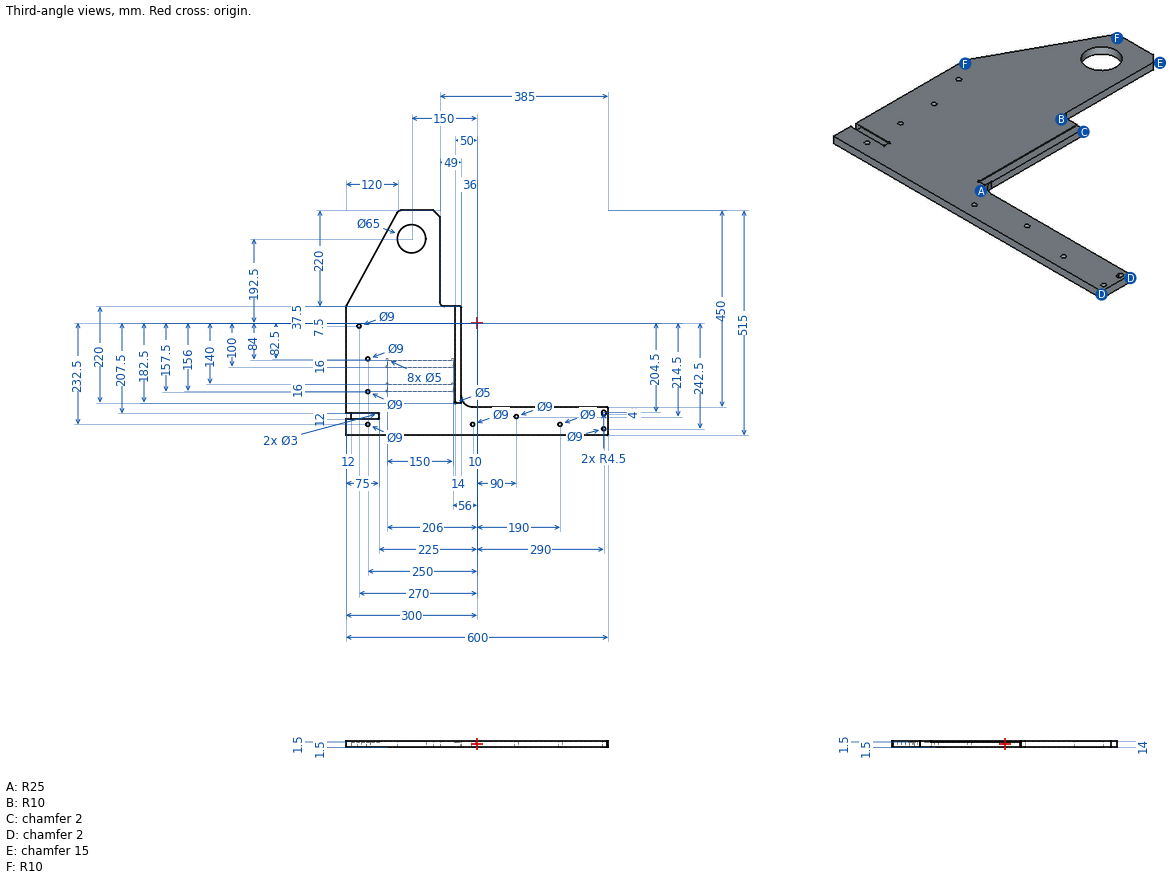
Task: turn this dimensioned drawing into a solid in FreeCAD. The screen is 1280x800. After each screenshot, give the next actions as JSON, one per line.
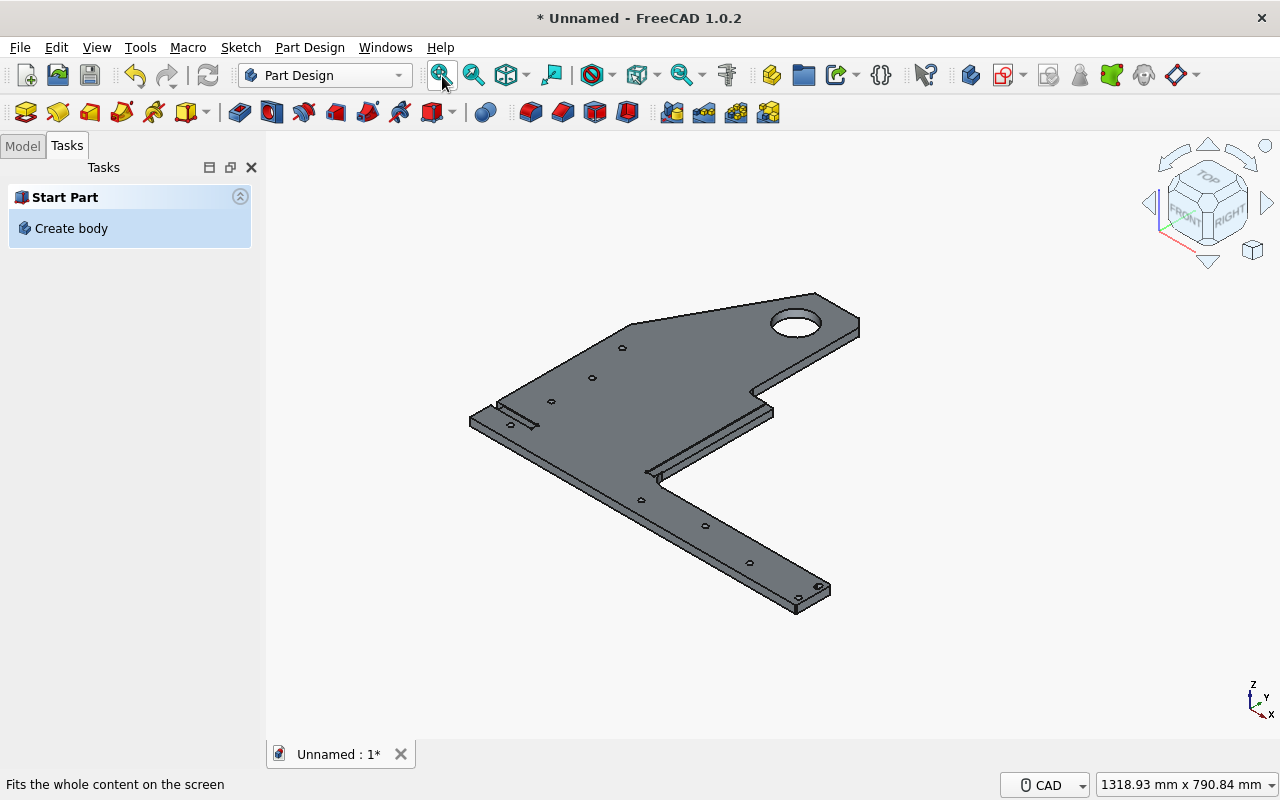
{"action": "key", "text": "2"}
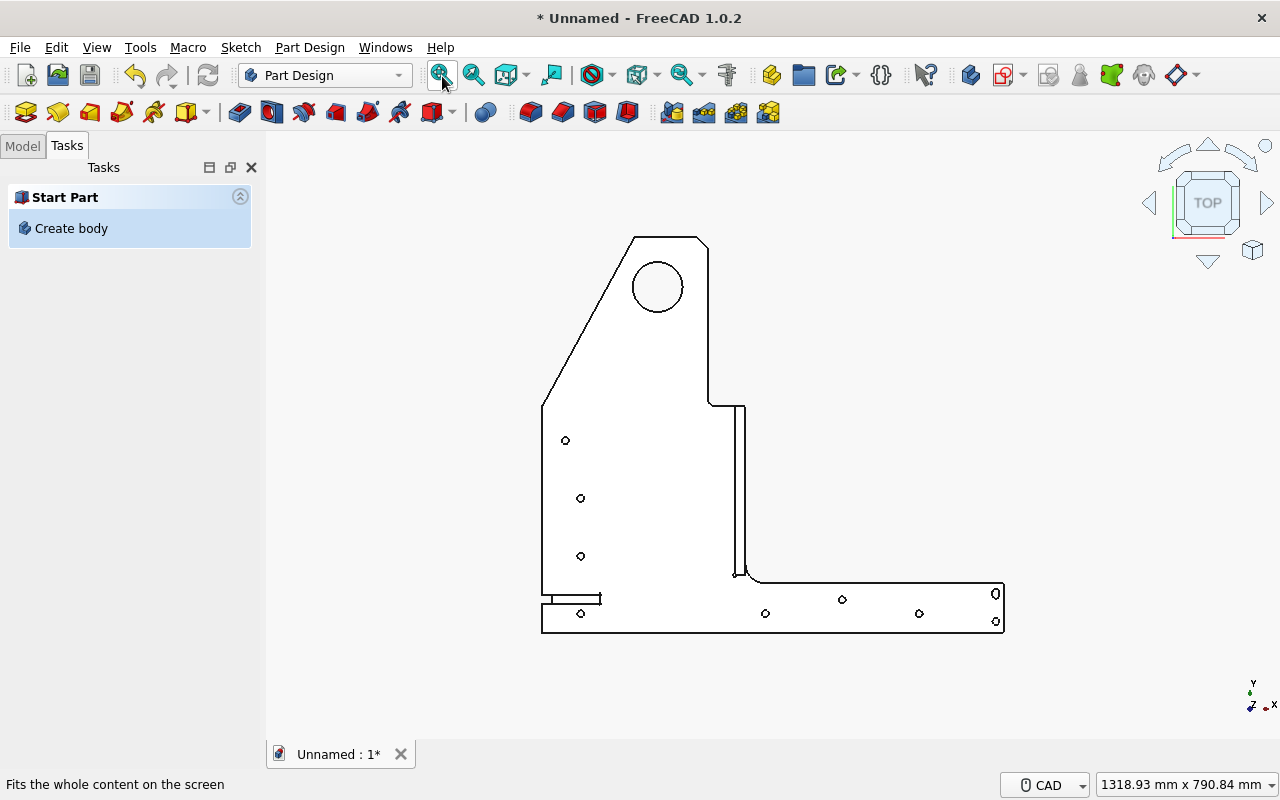
{"action": "scroll", "coordinate": [635, 236], "scroll_direction": "up", "scroll_amount": 7}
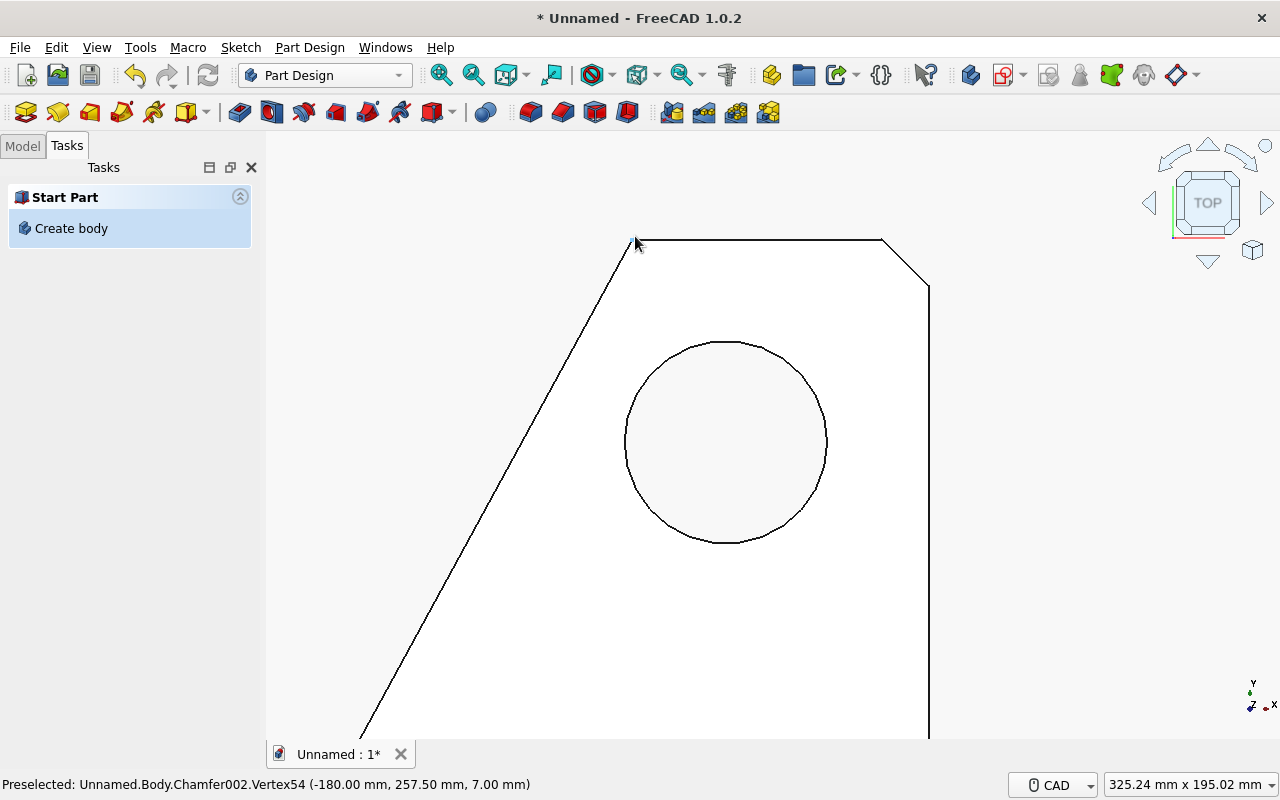
{"action": "left_click", "coordinate": [442, 76]}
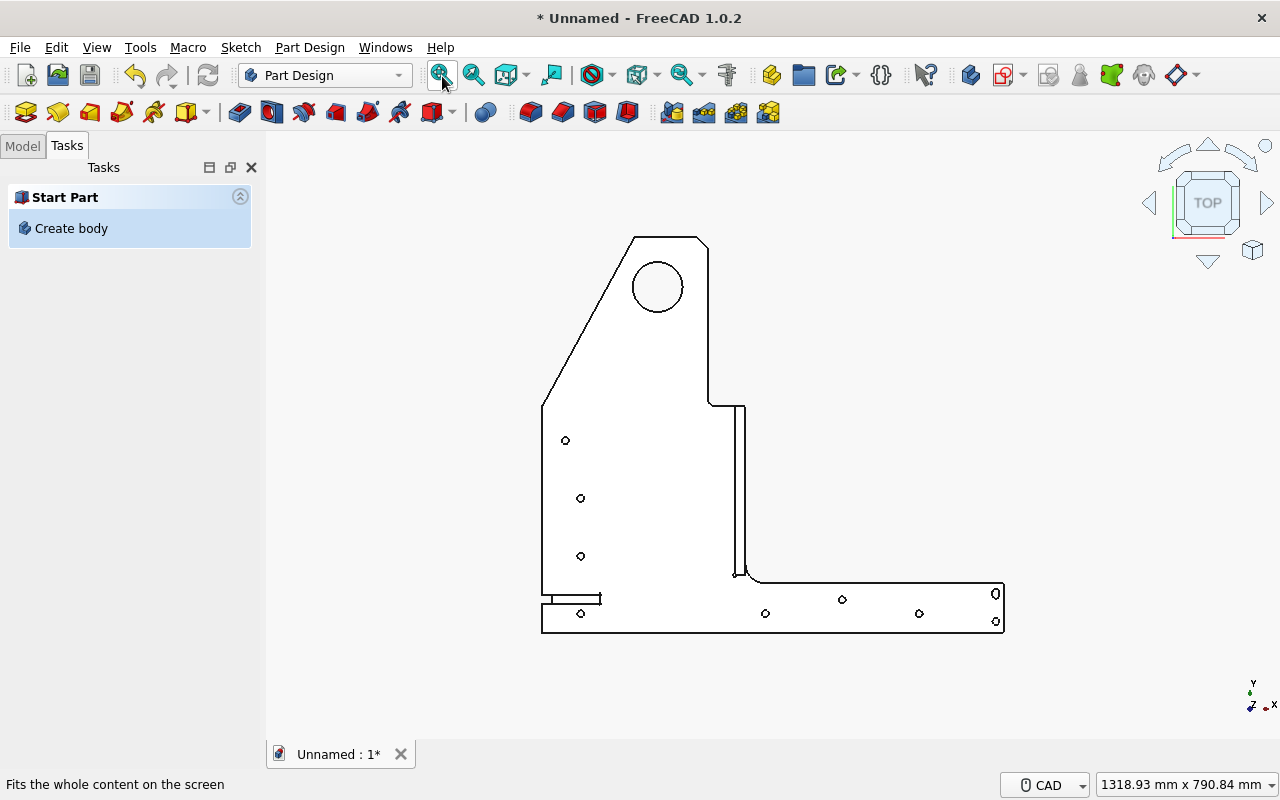
{"action": "key", "text": "1"}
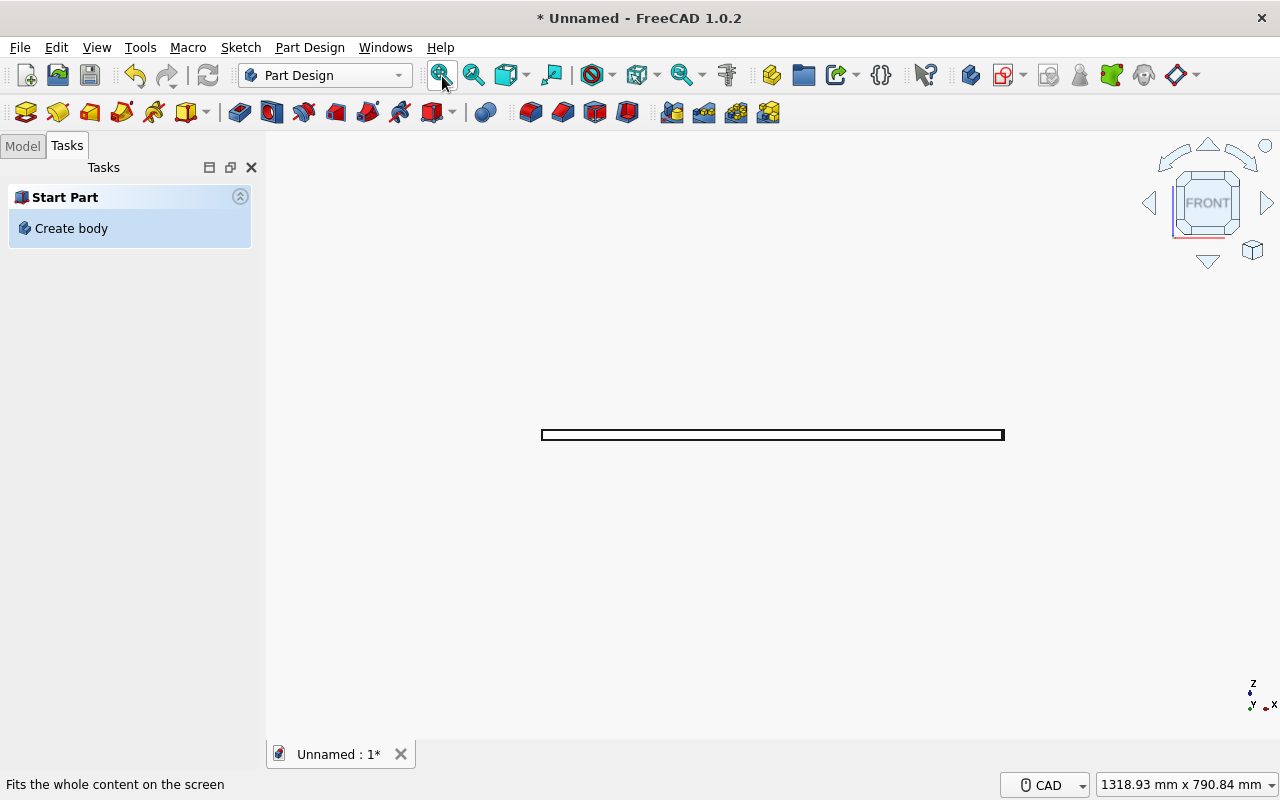
{"action": "scroll", "coordinate": [635, 434], "scroll_direction": "up", "scroll_amount": 7}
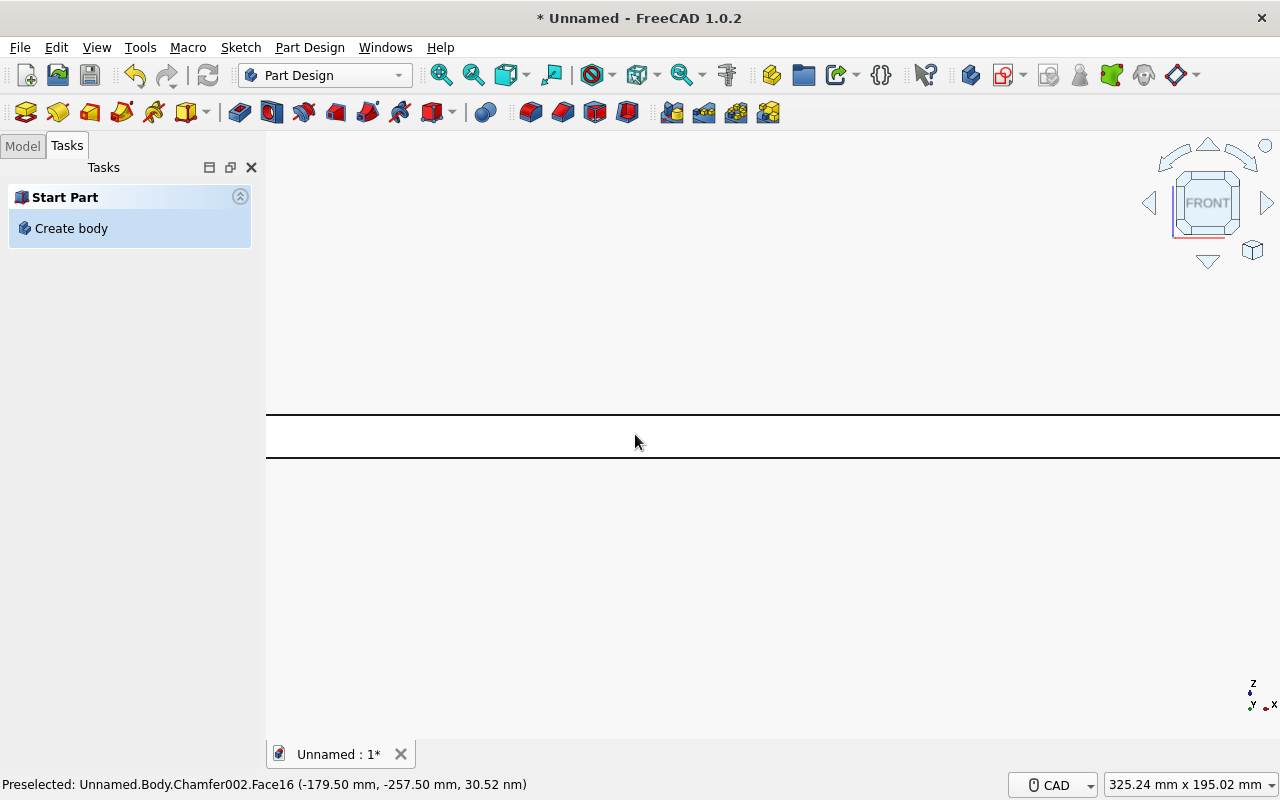
{"action": "left_click", "coordinate": [442, 76]}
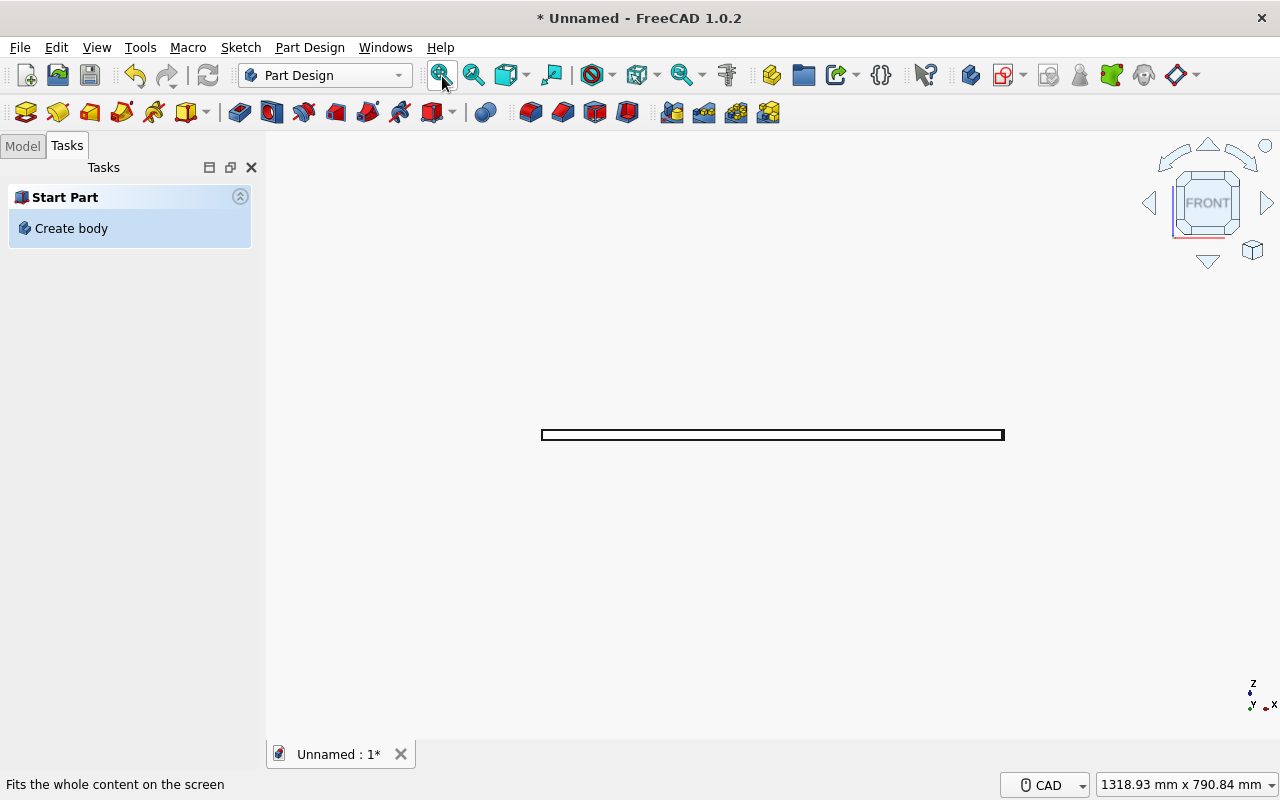
{"action": "key", "text": "3"}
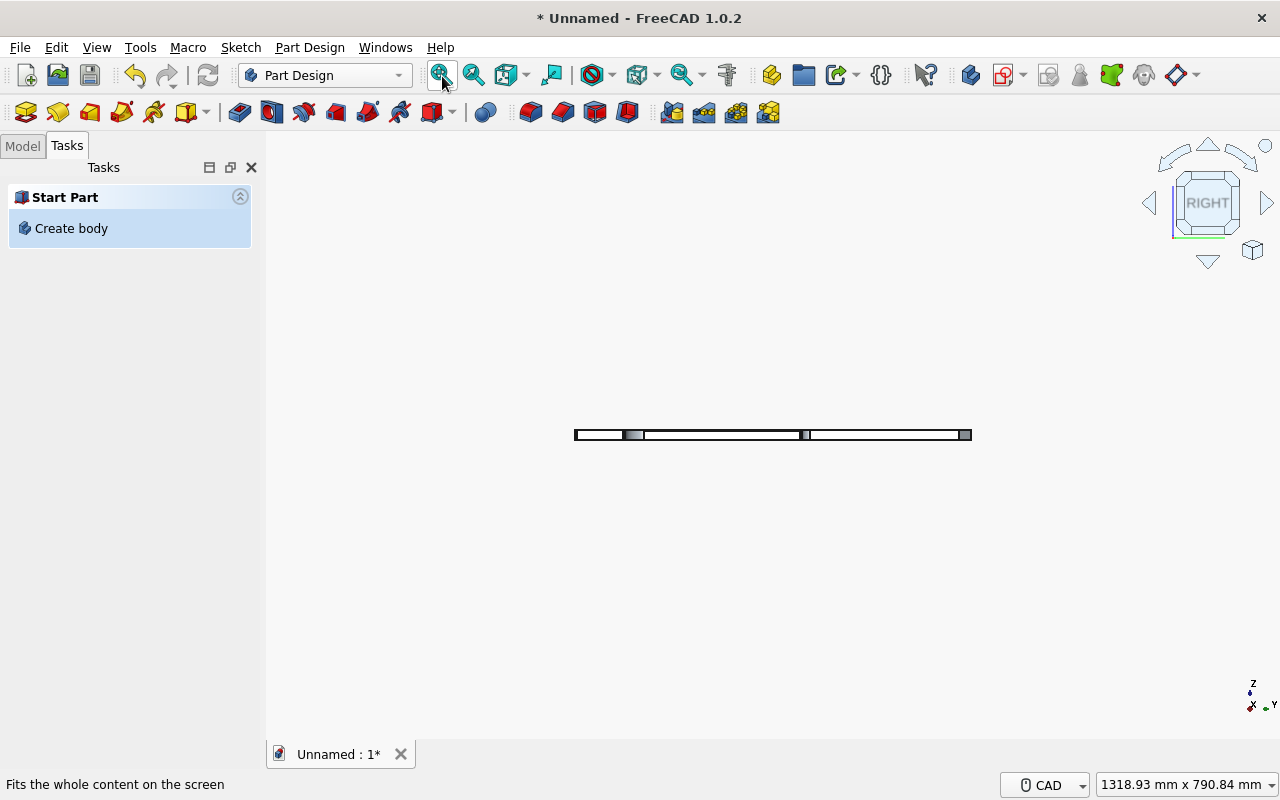
{"action": "left_click", "coordinate": [442, 76]}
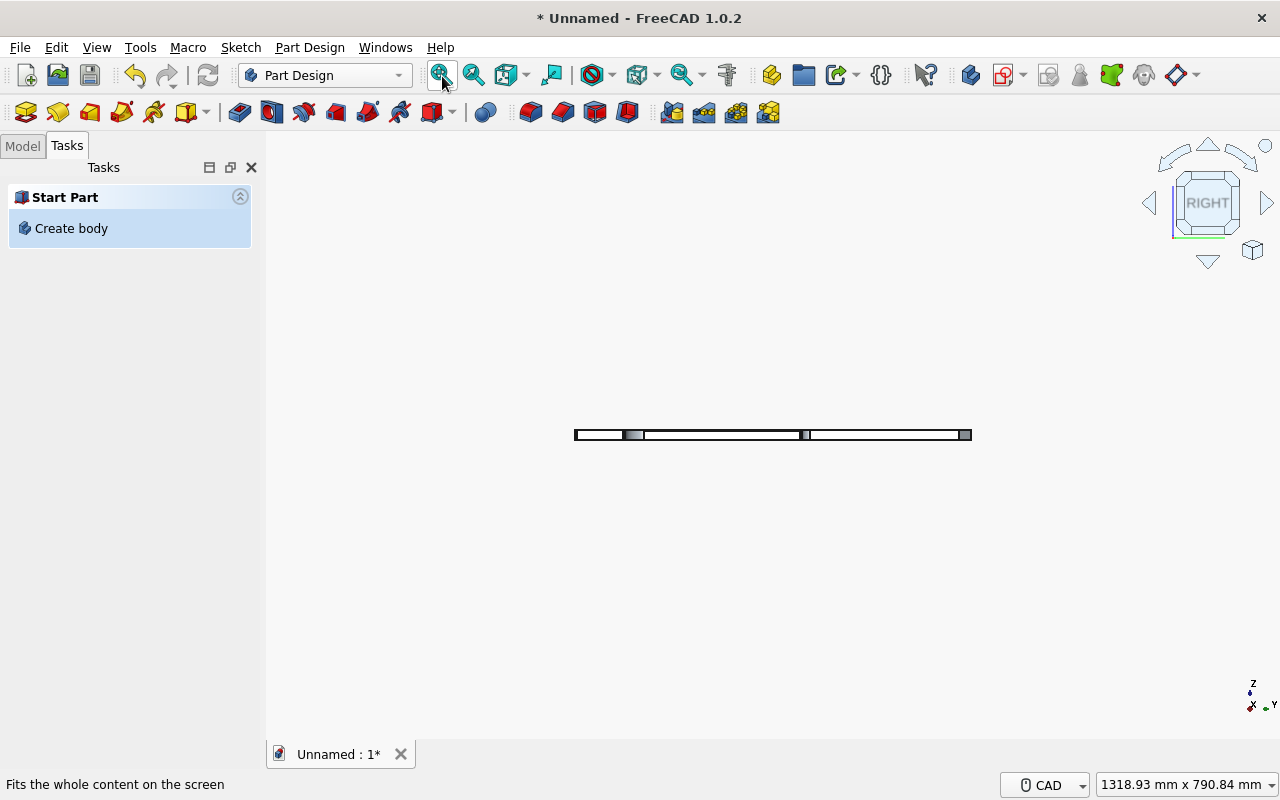
{"action": "scroll", "coordinate": [971, 434], "scroll_direction": "up", "scroll_amount": 7}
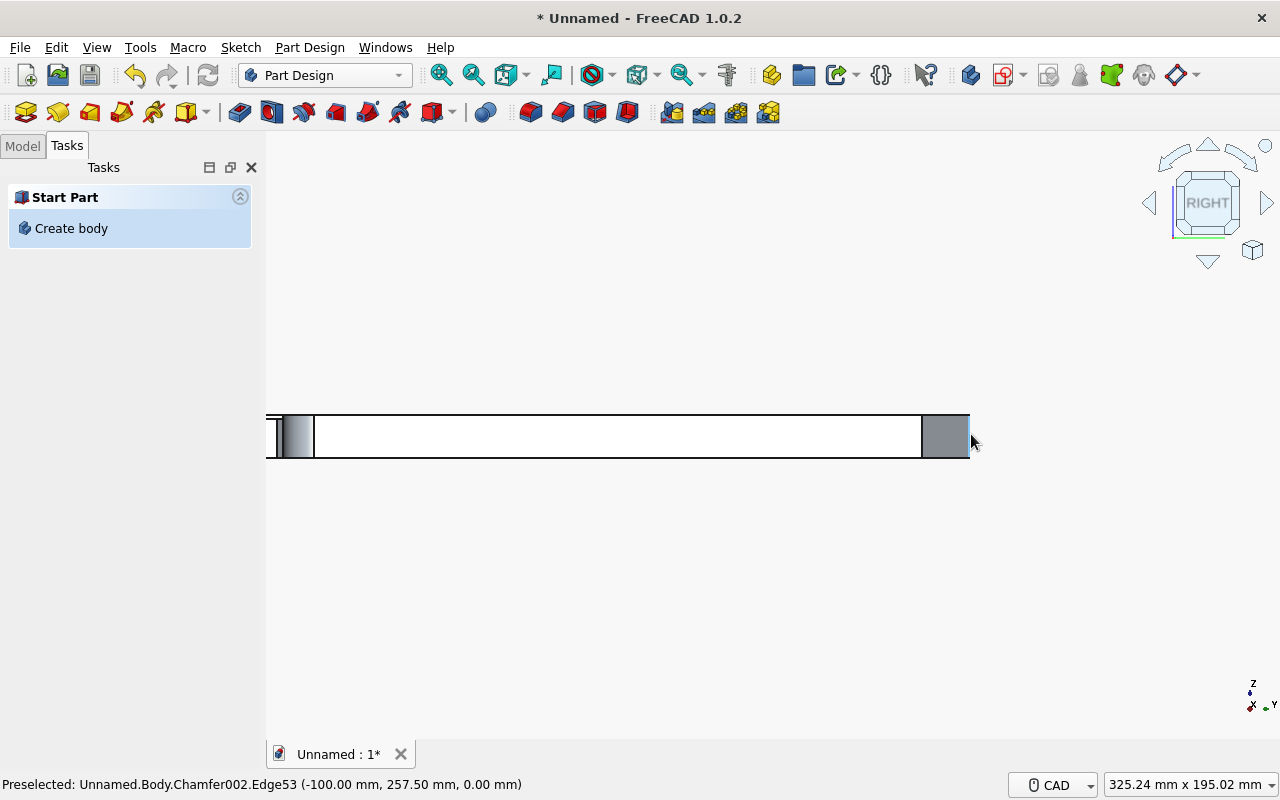
{"action": "left_click", "coordinate": [442, 76]}